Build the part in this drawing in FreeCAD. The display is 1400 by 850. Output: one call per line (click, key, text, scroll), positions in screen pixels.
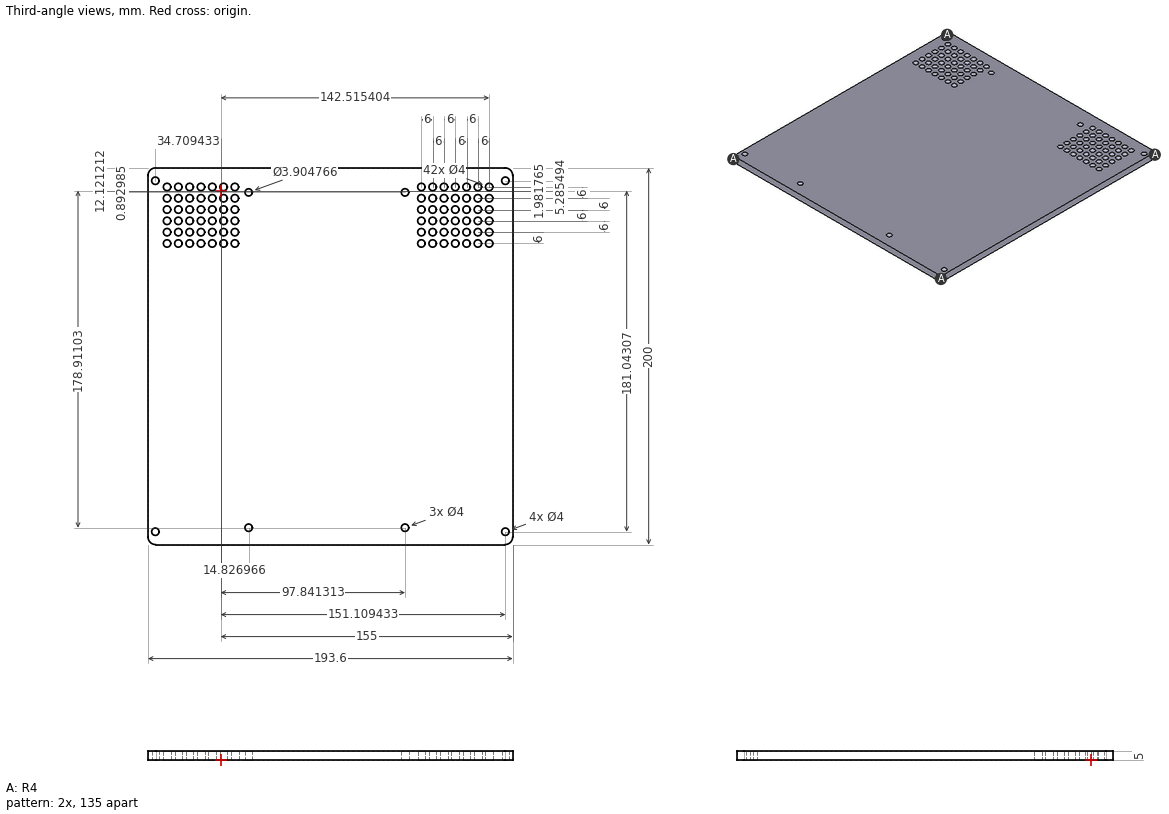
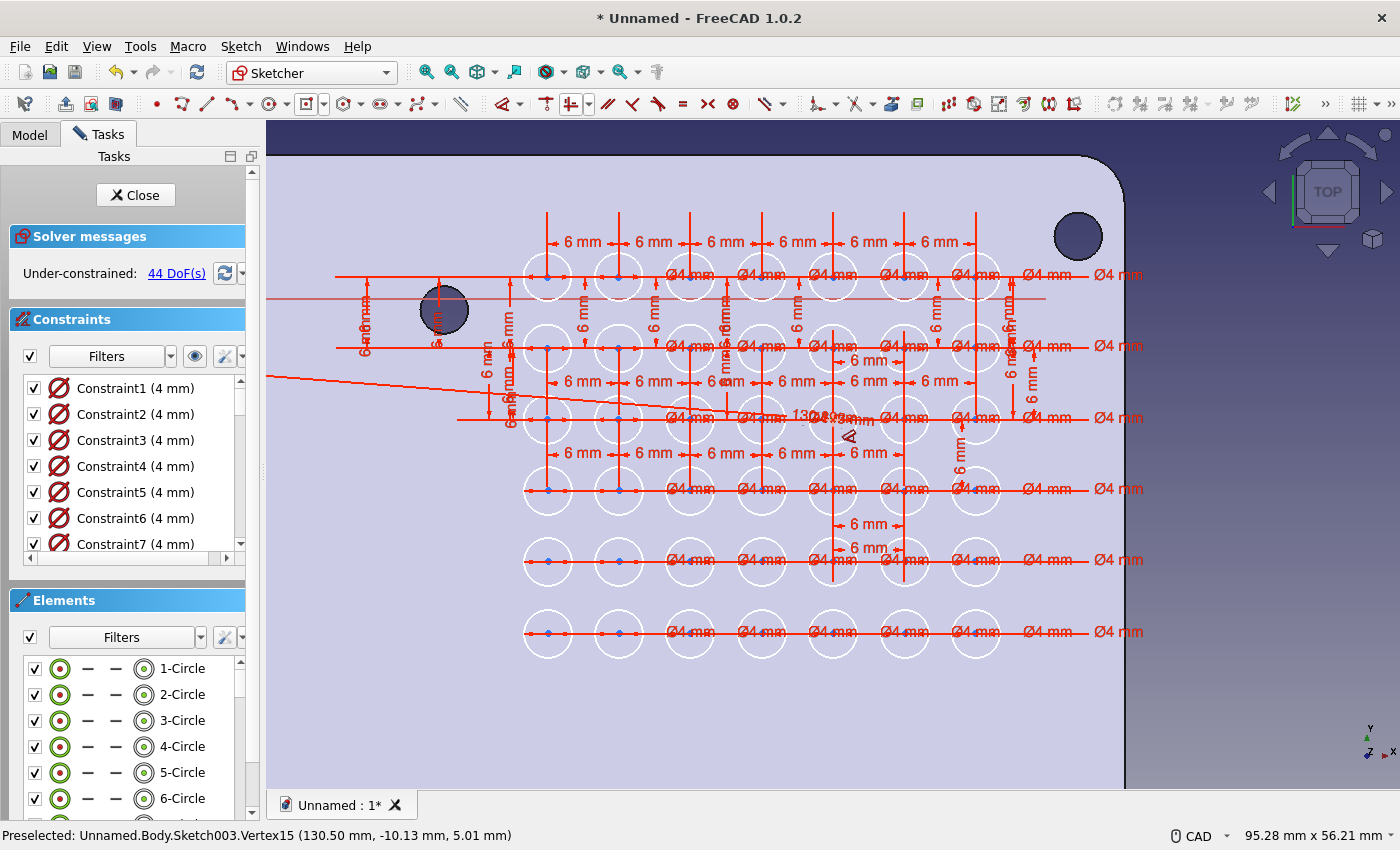
click(833, 491)
click(1013, 431)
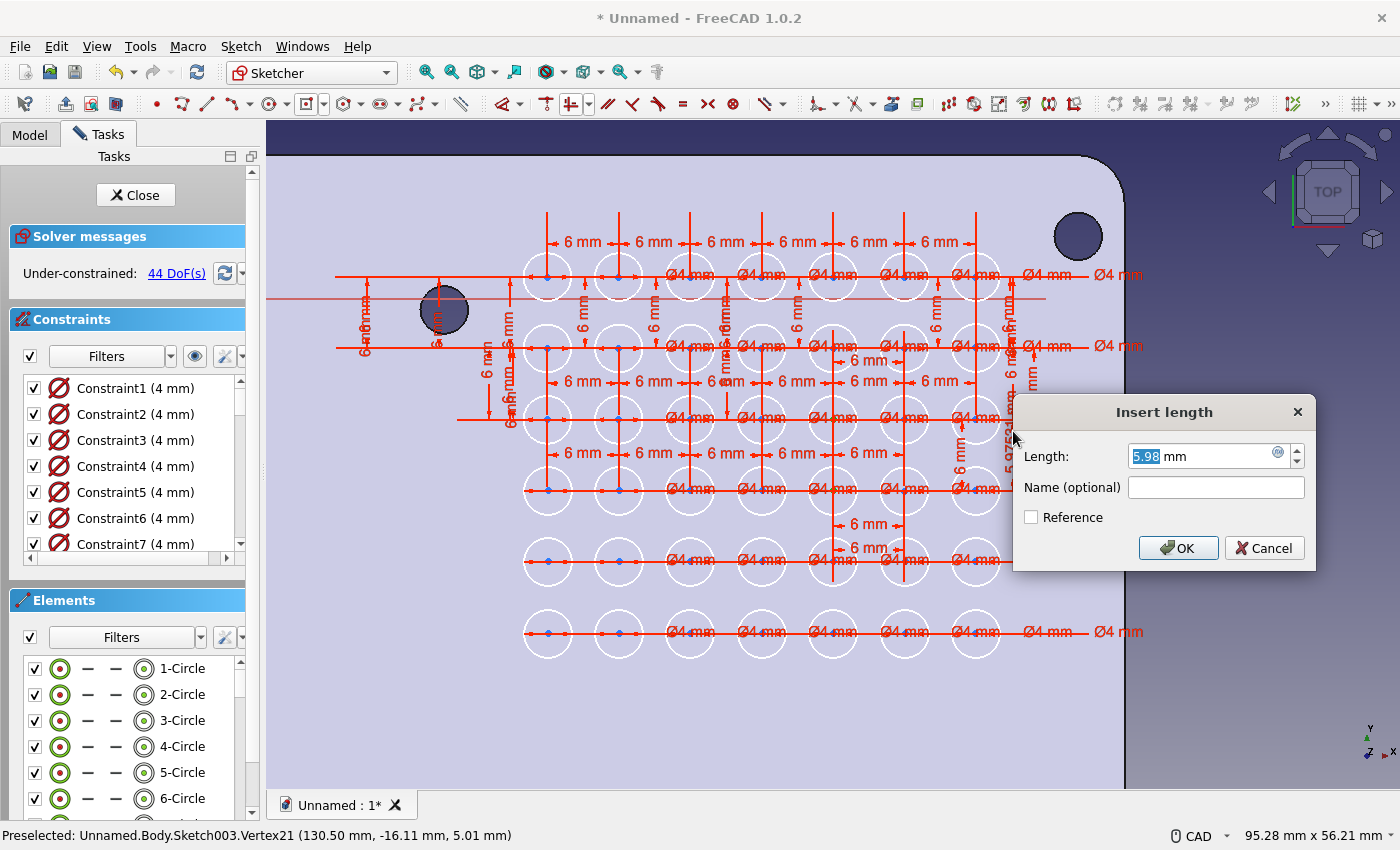
text(6)
key(Return)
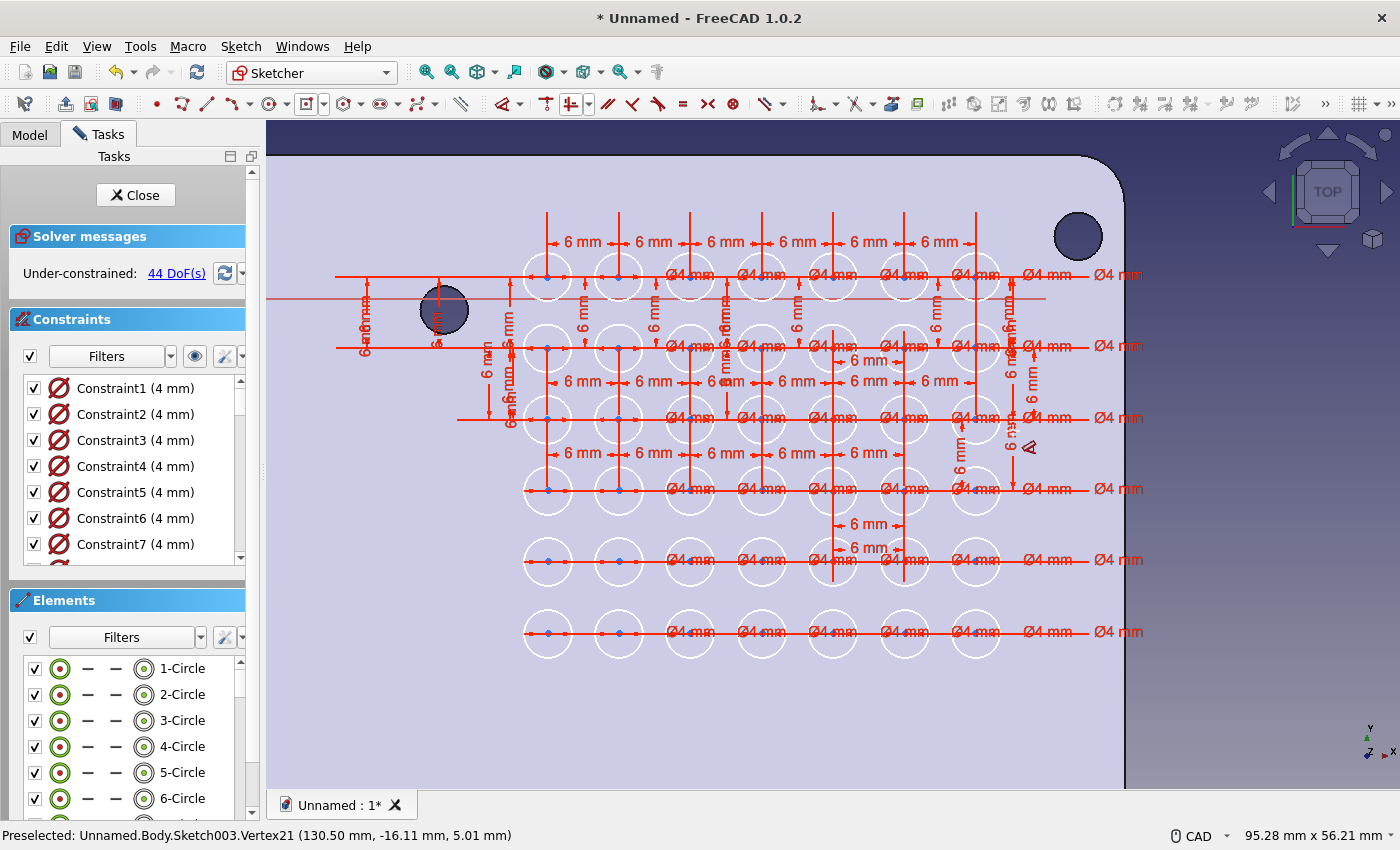
click(833, 491)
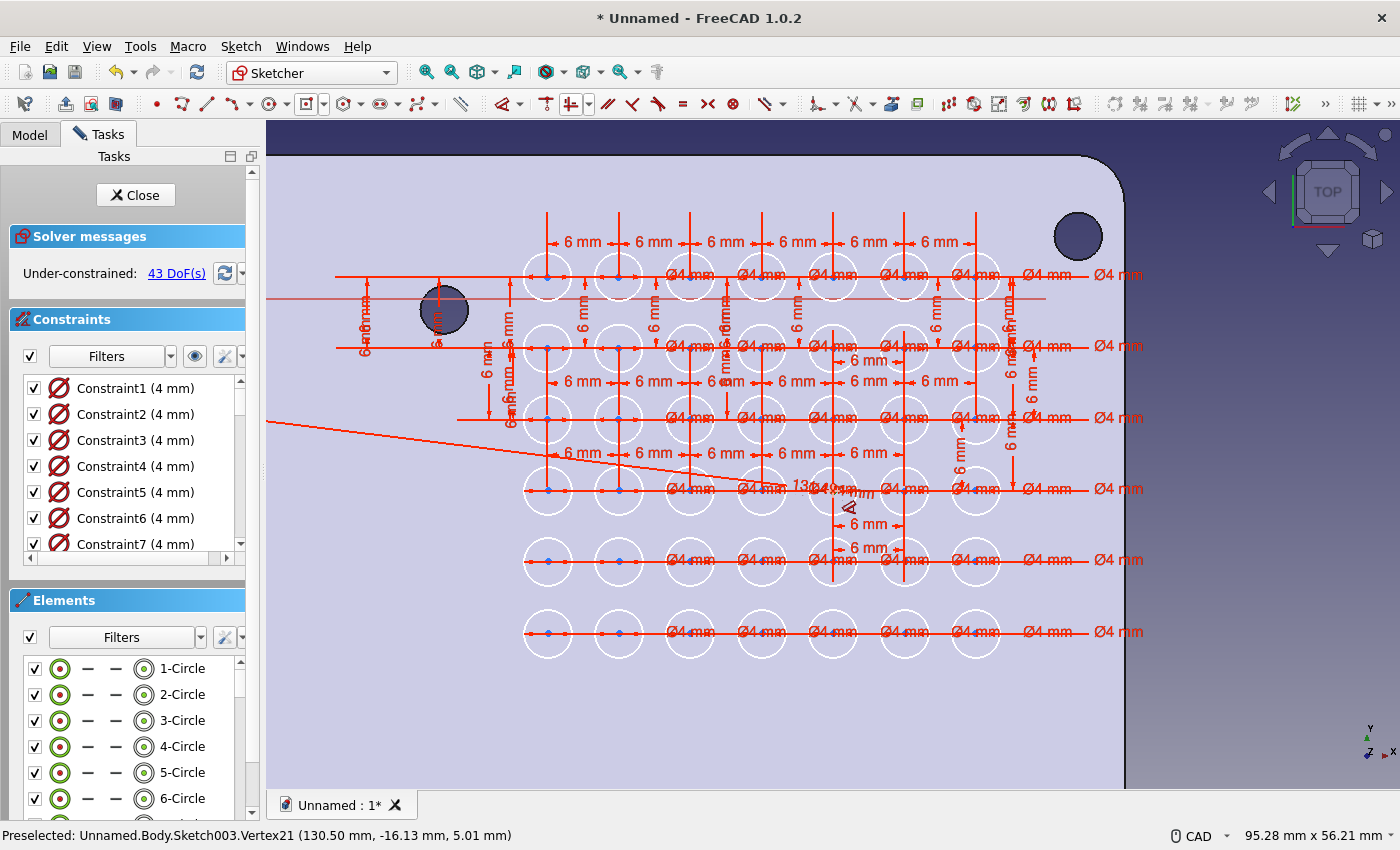
click(762, 491)
click(798, 525)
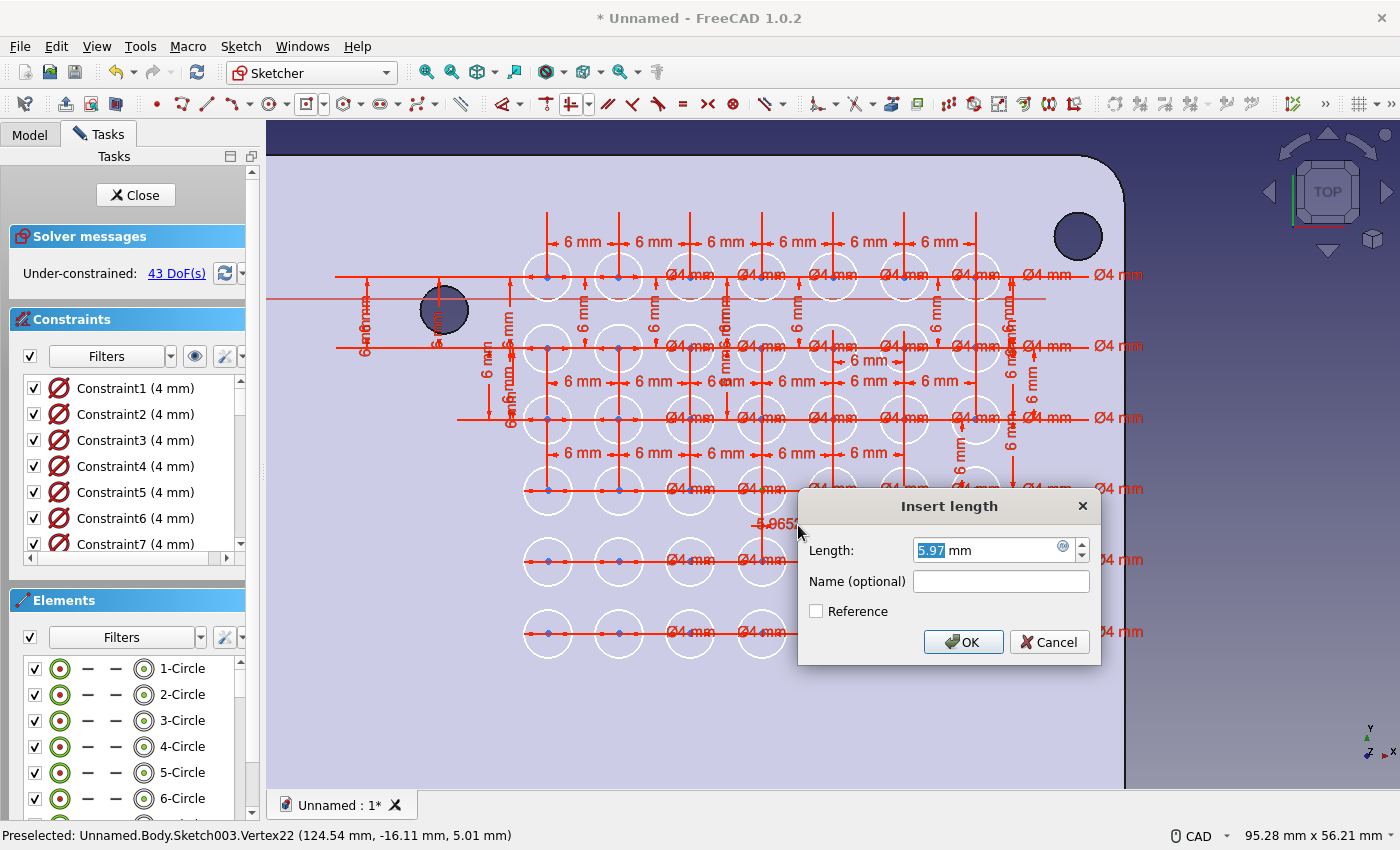
text(6)
key(Return)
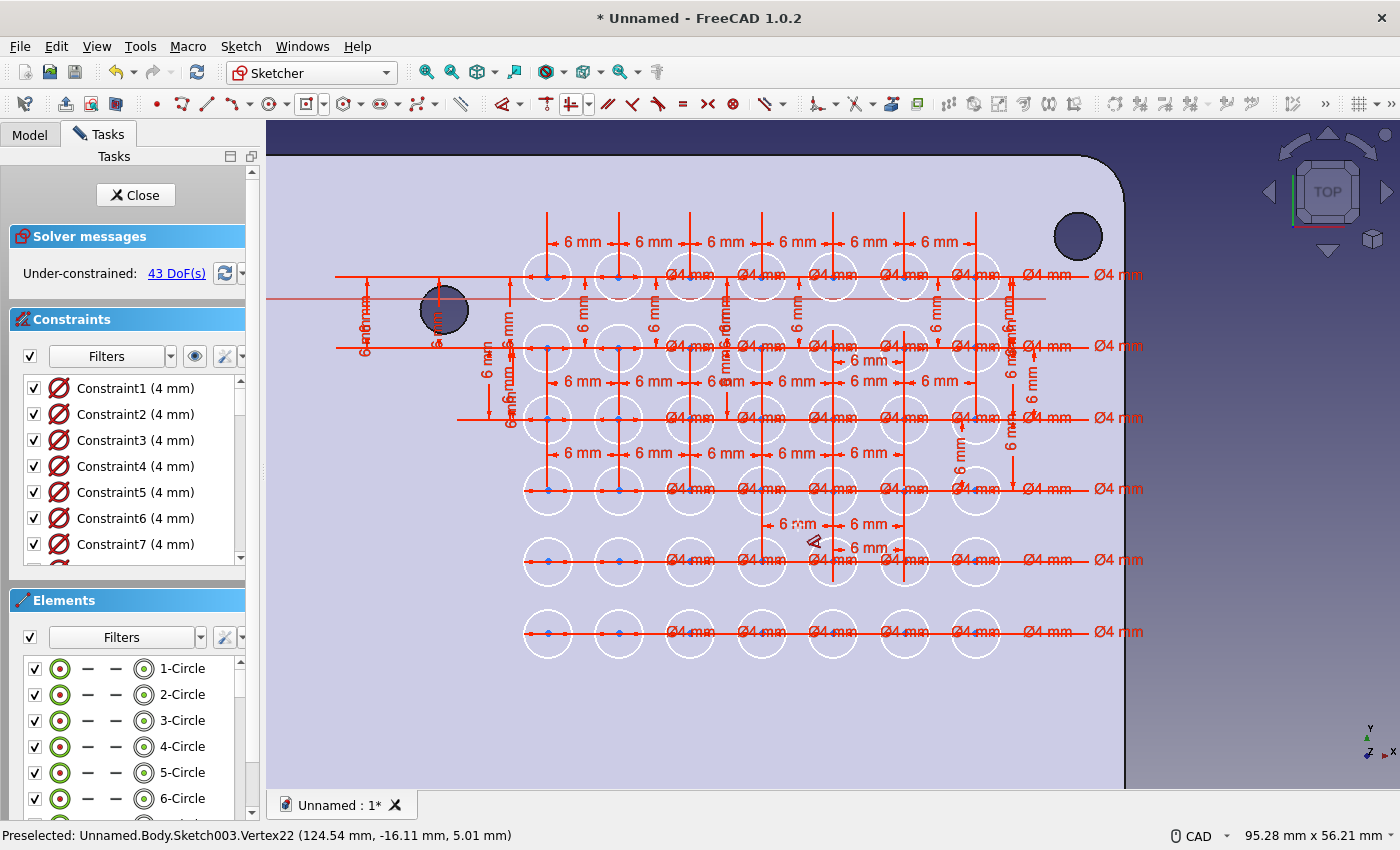
click(762, 420)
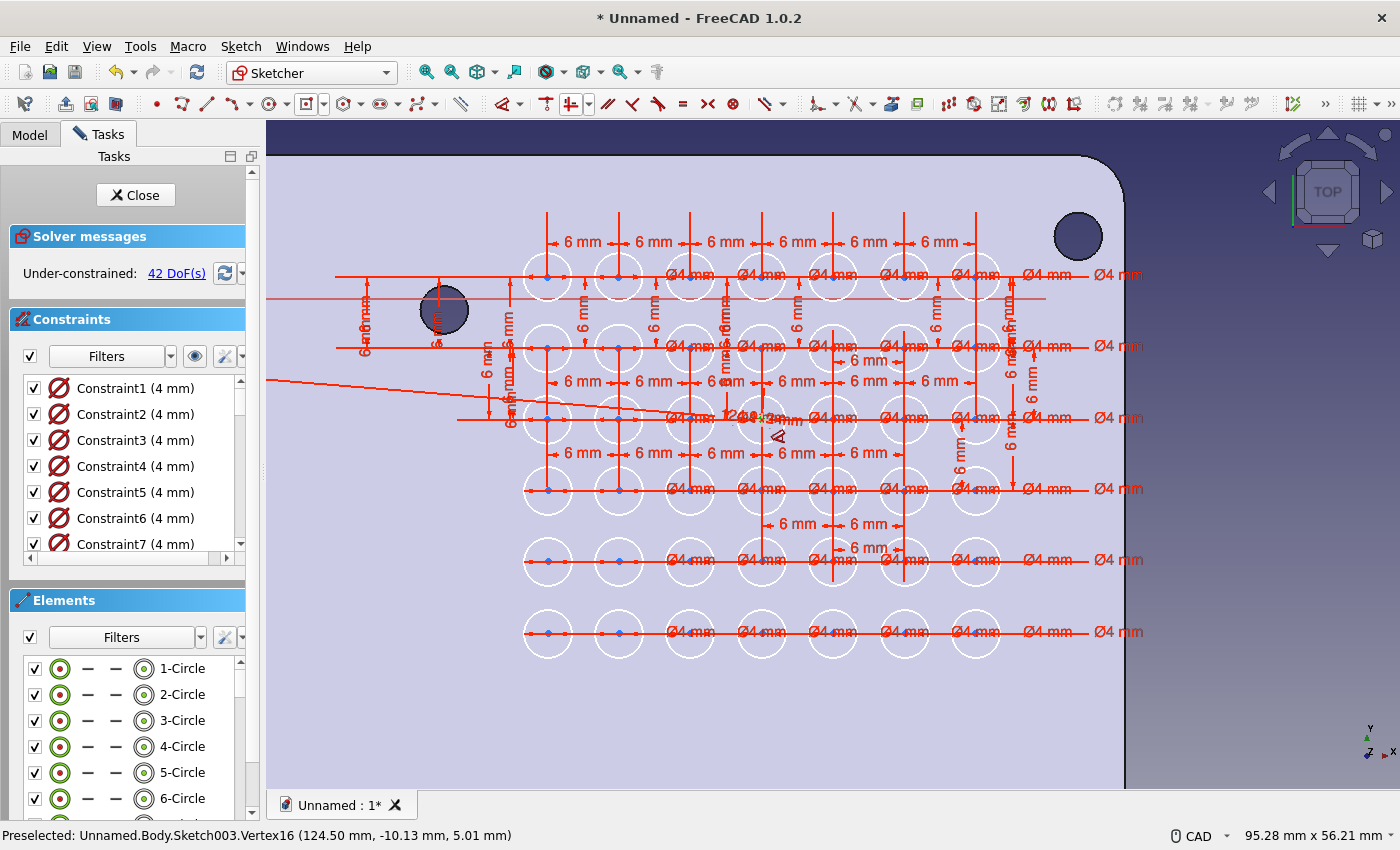
click(762, 491)
click(728, 439)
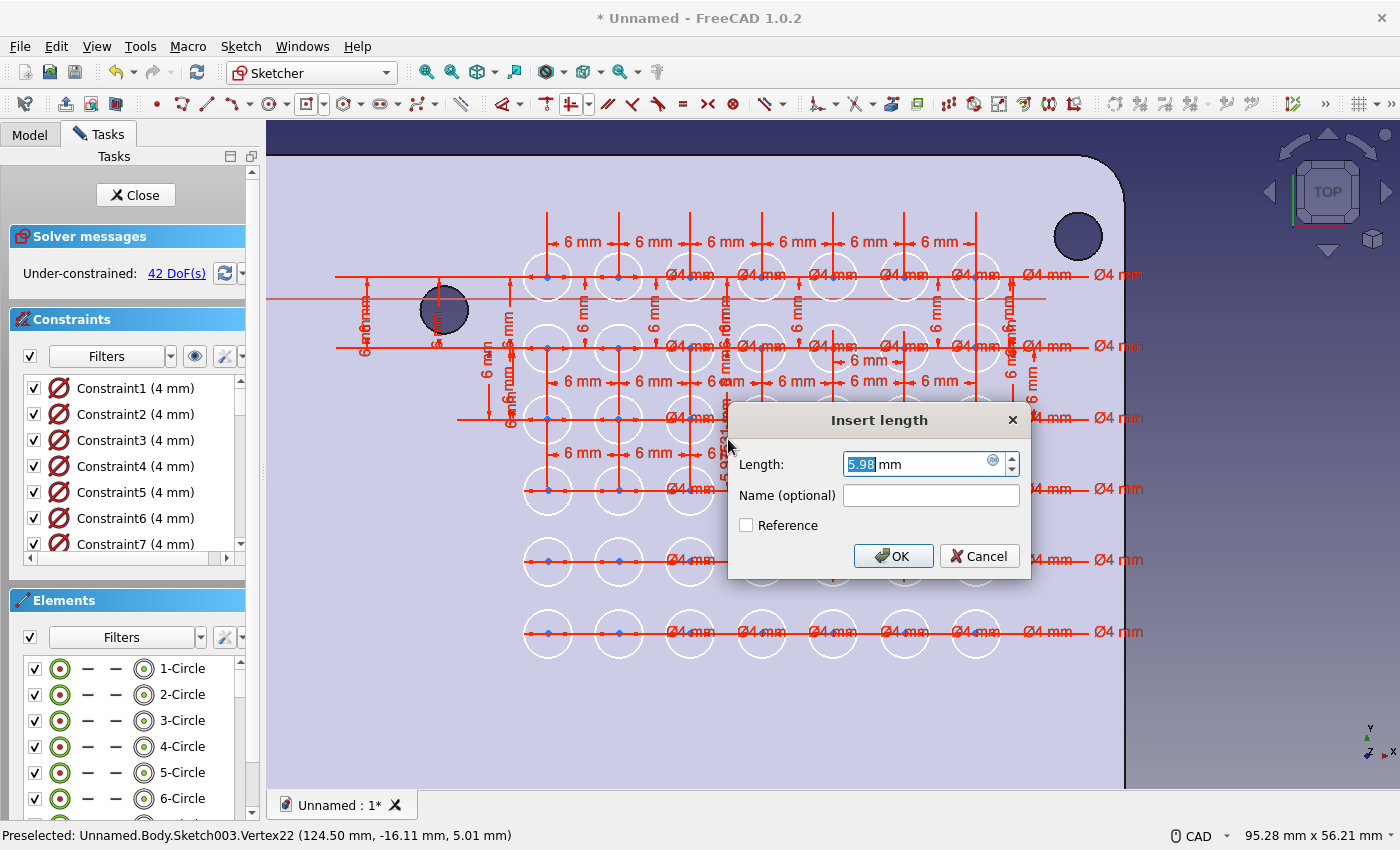
text(6)
key(Return)